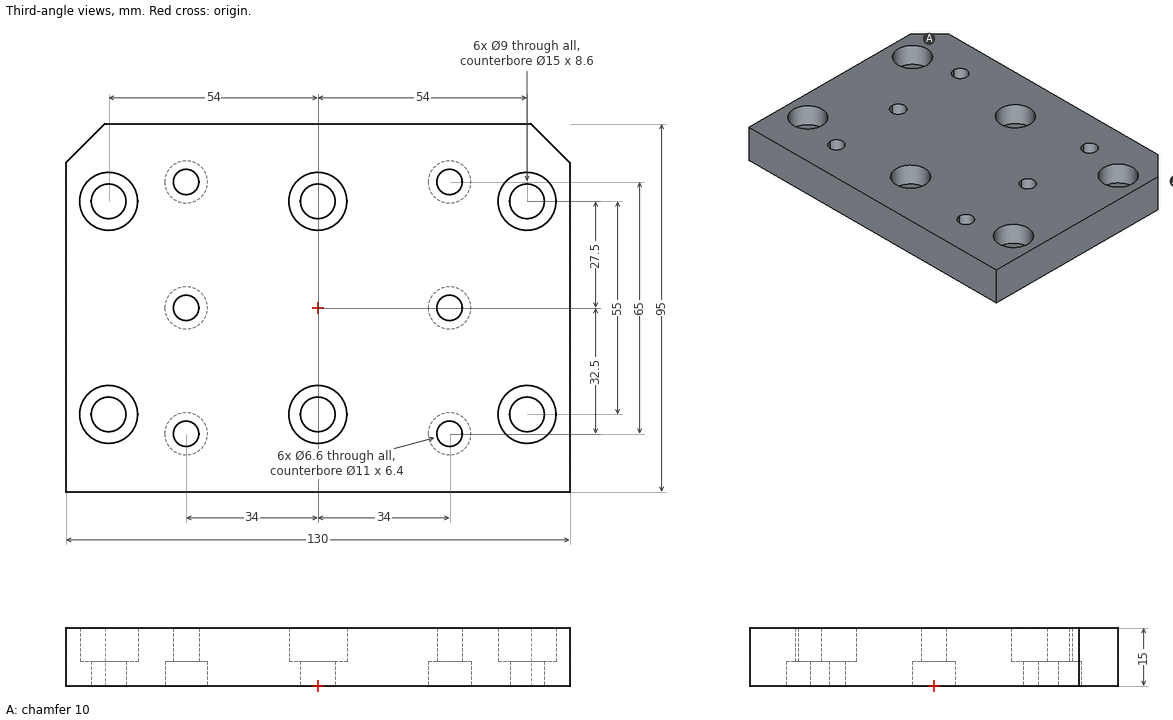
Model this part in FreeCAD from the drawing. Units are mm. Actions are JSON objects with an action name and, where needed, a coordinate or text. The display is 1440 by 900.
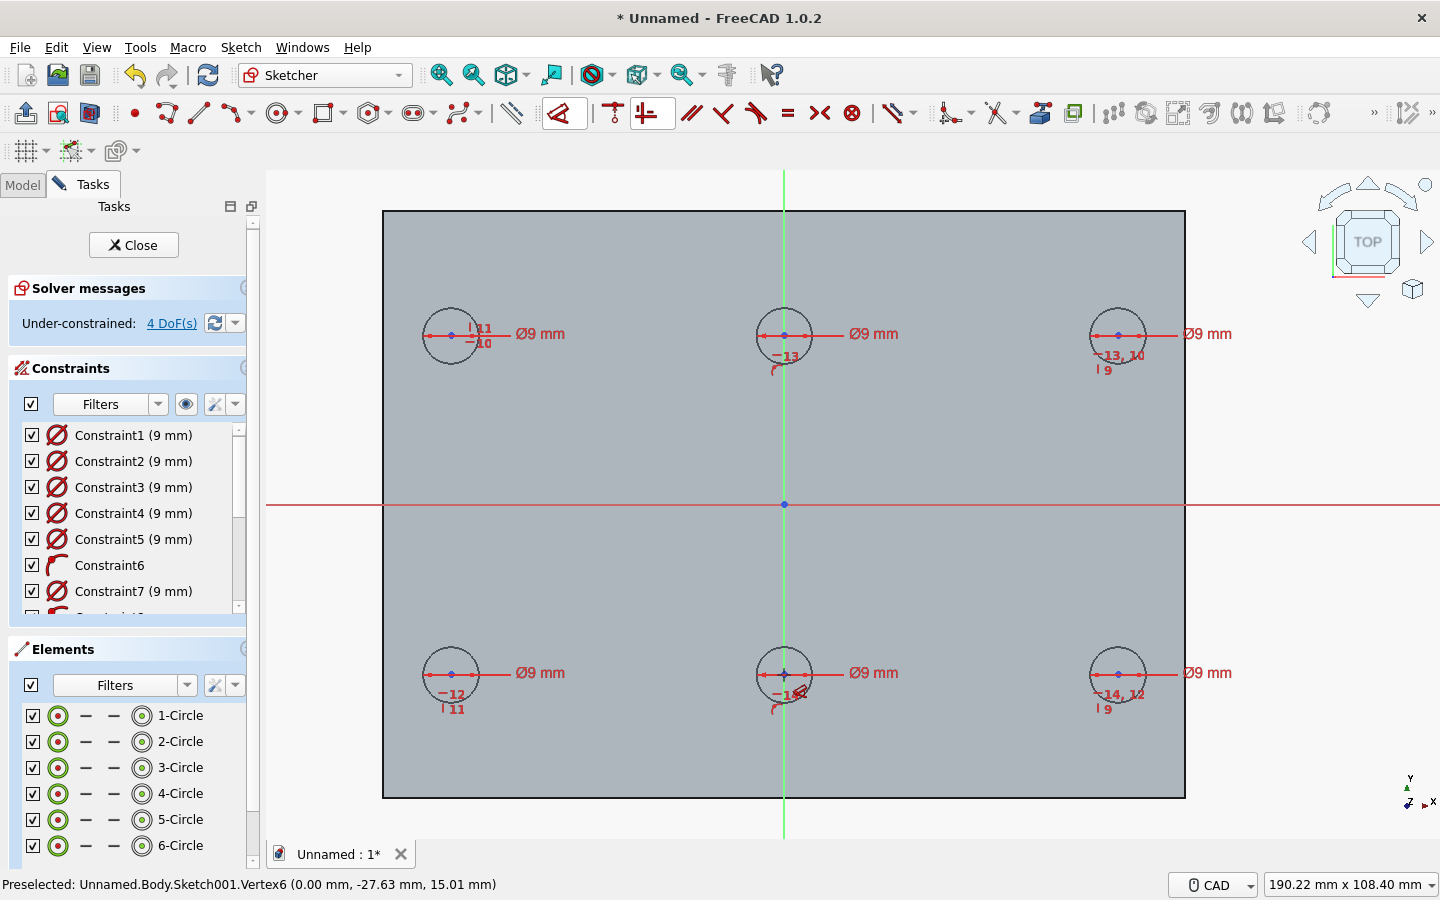
{"action": "left_click", "coordinate": [1118, 336]}
{"action": "left_click", "coordinate": [951, 302]}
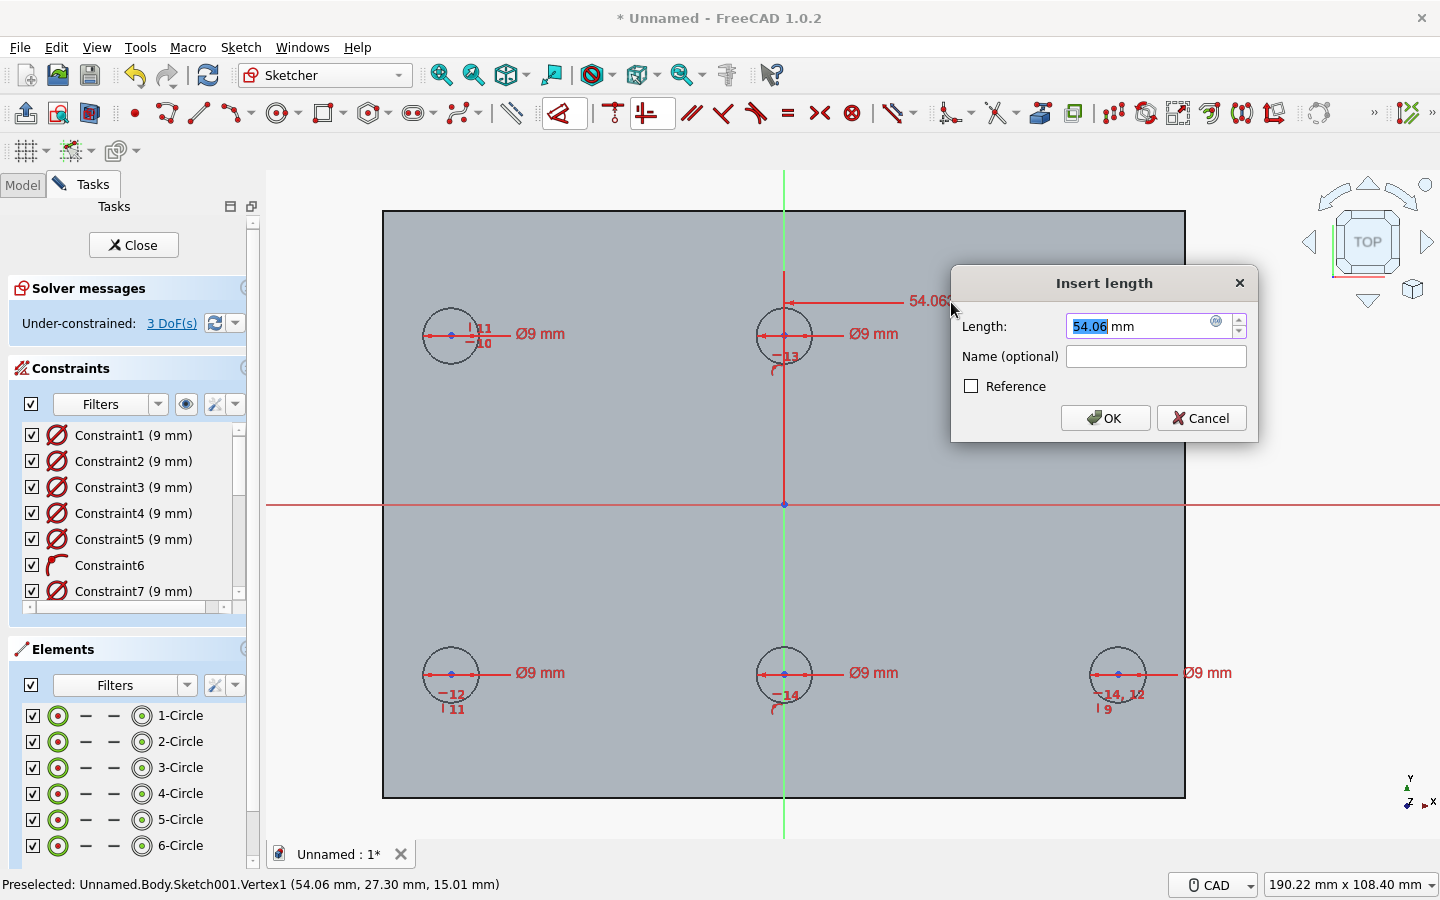
{"action": "type", "text": "54"}
{"action": "key", "text": "Return"}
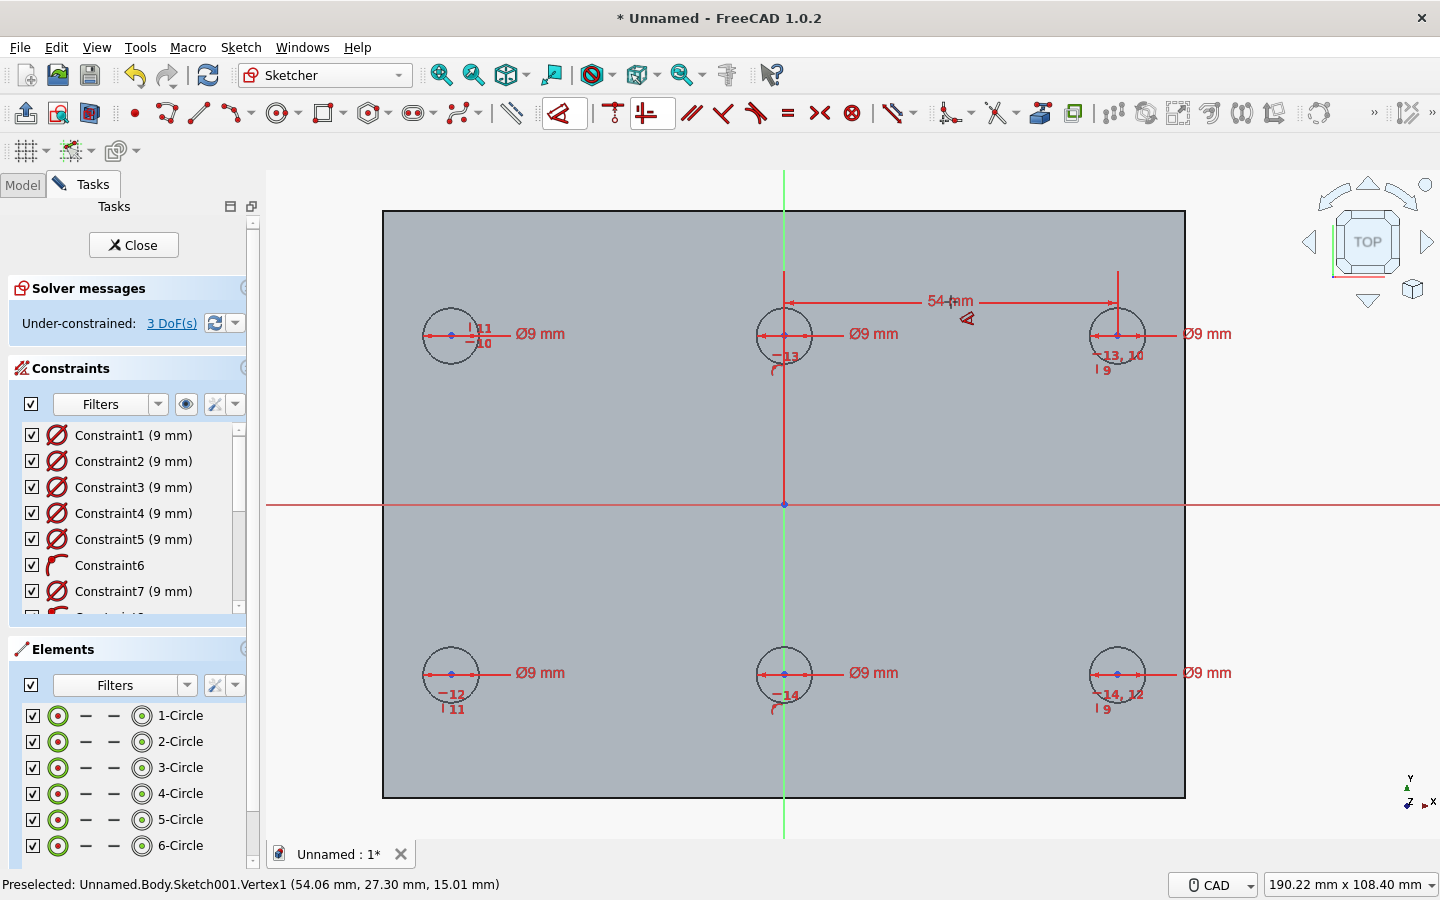
{"action": "left_click", "coordinate": [451, 336]}
{"action": "left_click", "coordinate": [618, 302]}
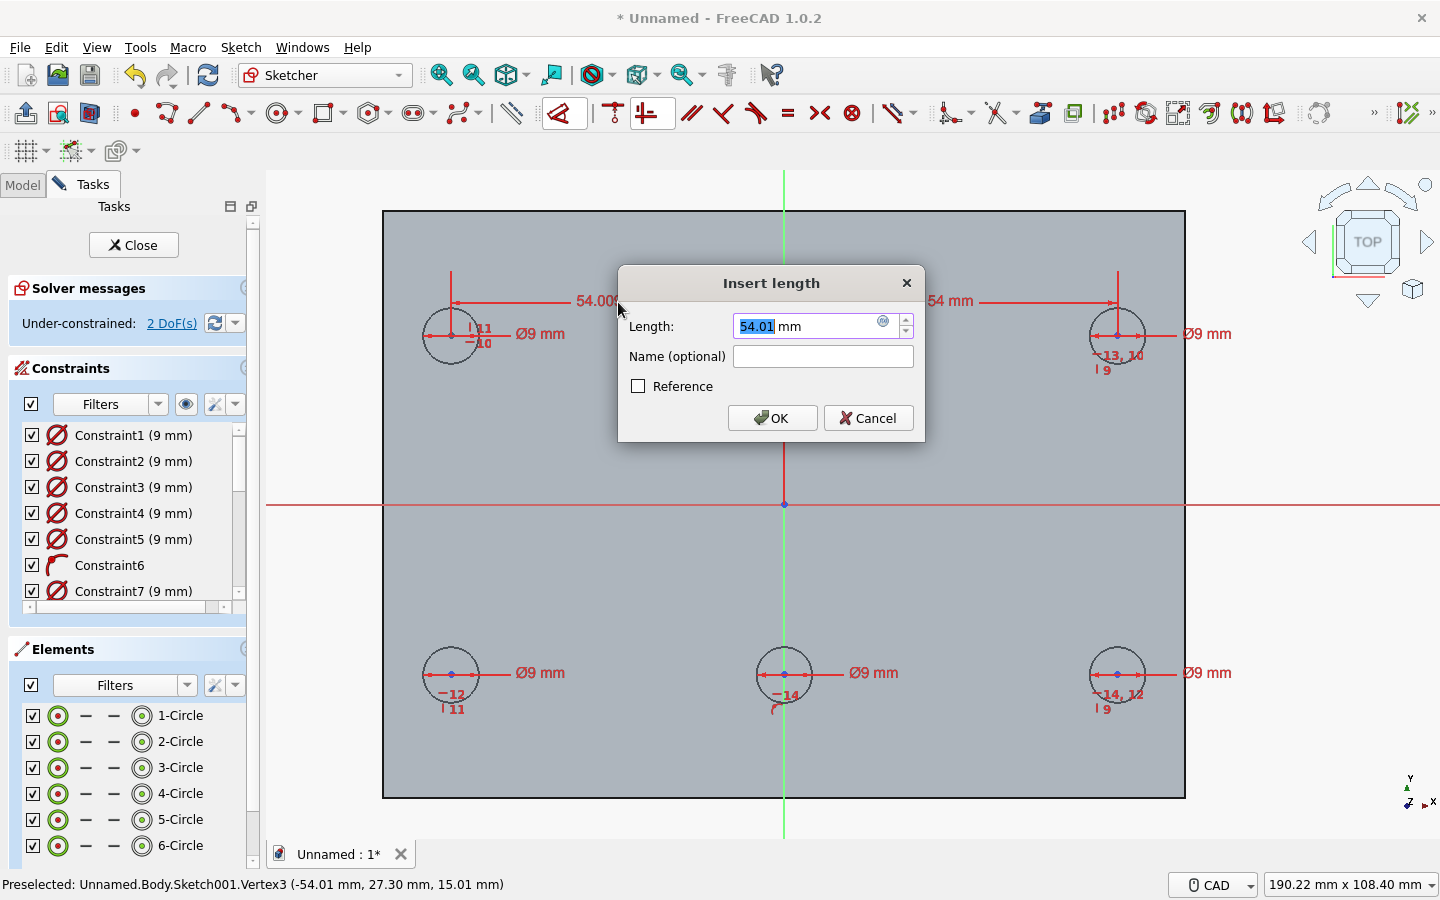
{"action": "type", "text": "54"}
{"action": "key", "text": "Return"}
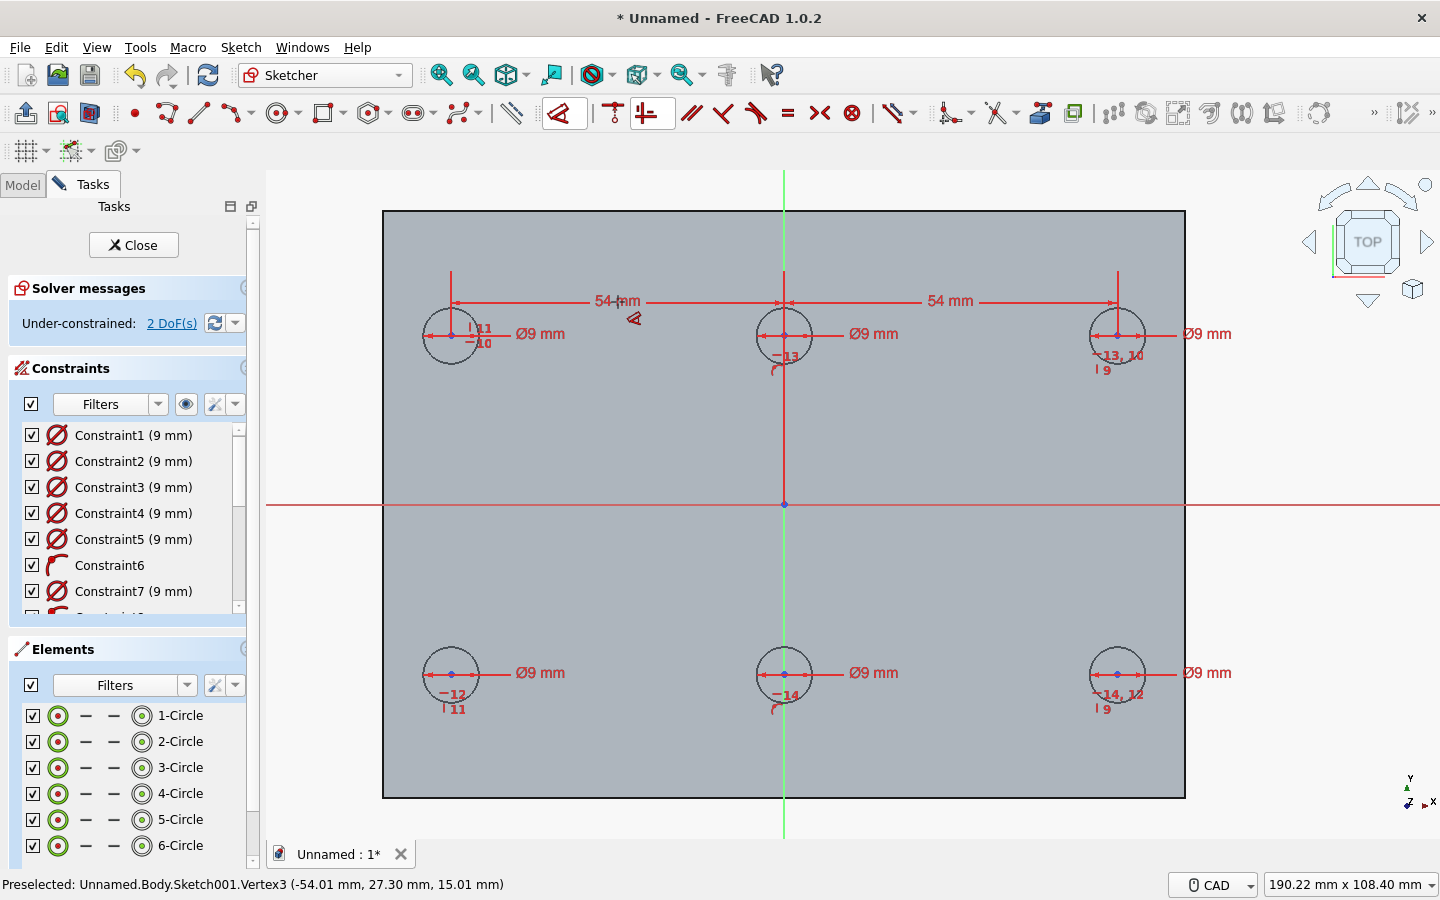
{"action": "left_click", "coordinate": [1118, 336]}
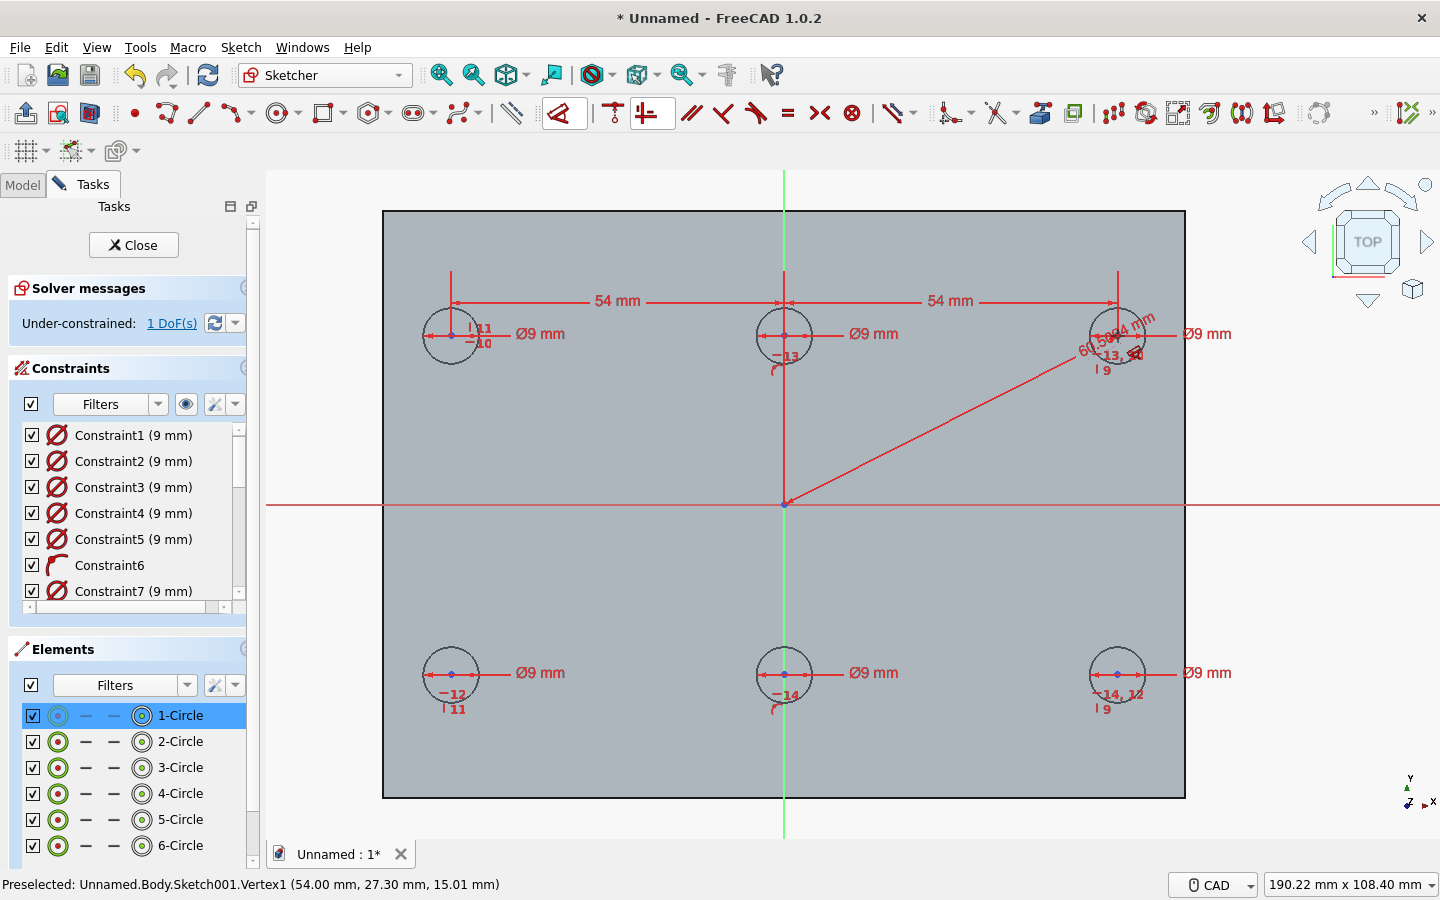
{"action": "left_click", "coordinate": [1118, 675]}
{"action": "left_click", "coordinate": [1152, 428]}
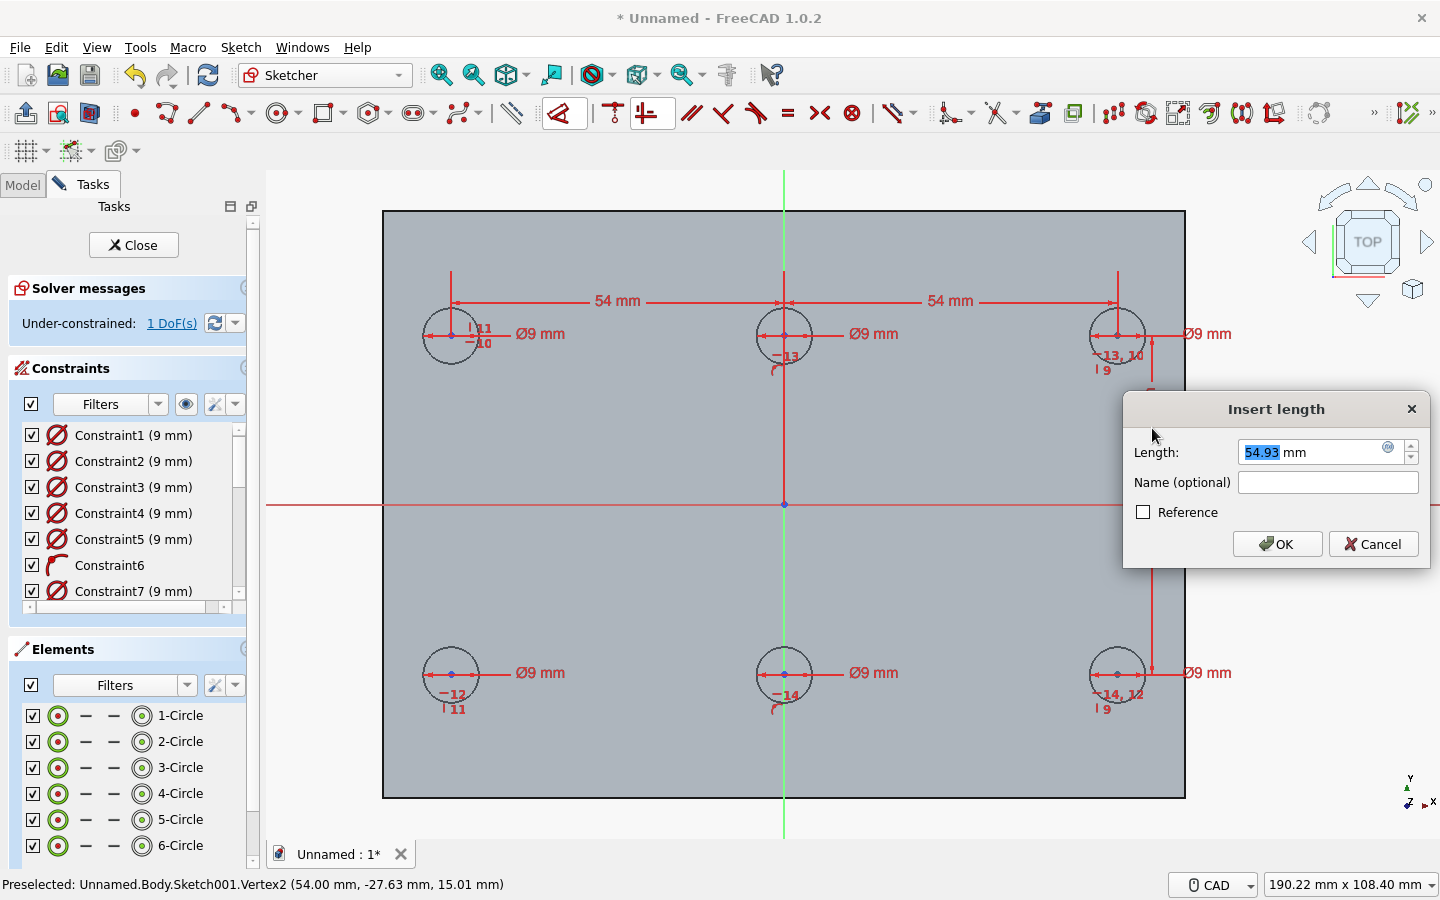
{"action": "type", "text": "55"}
{"action": "key", "text": "Return"}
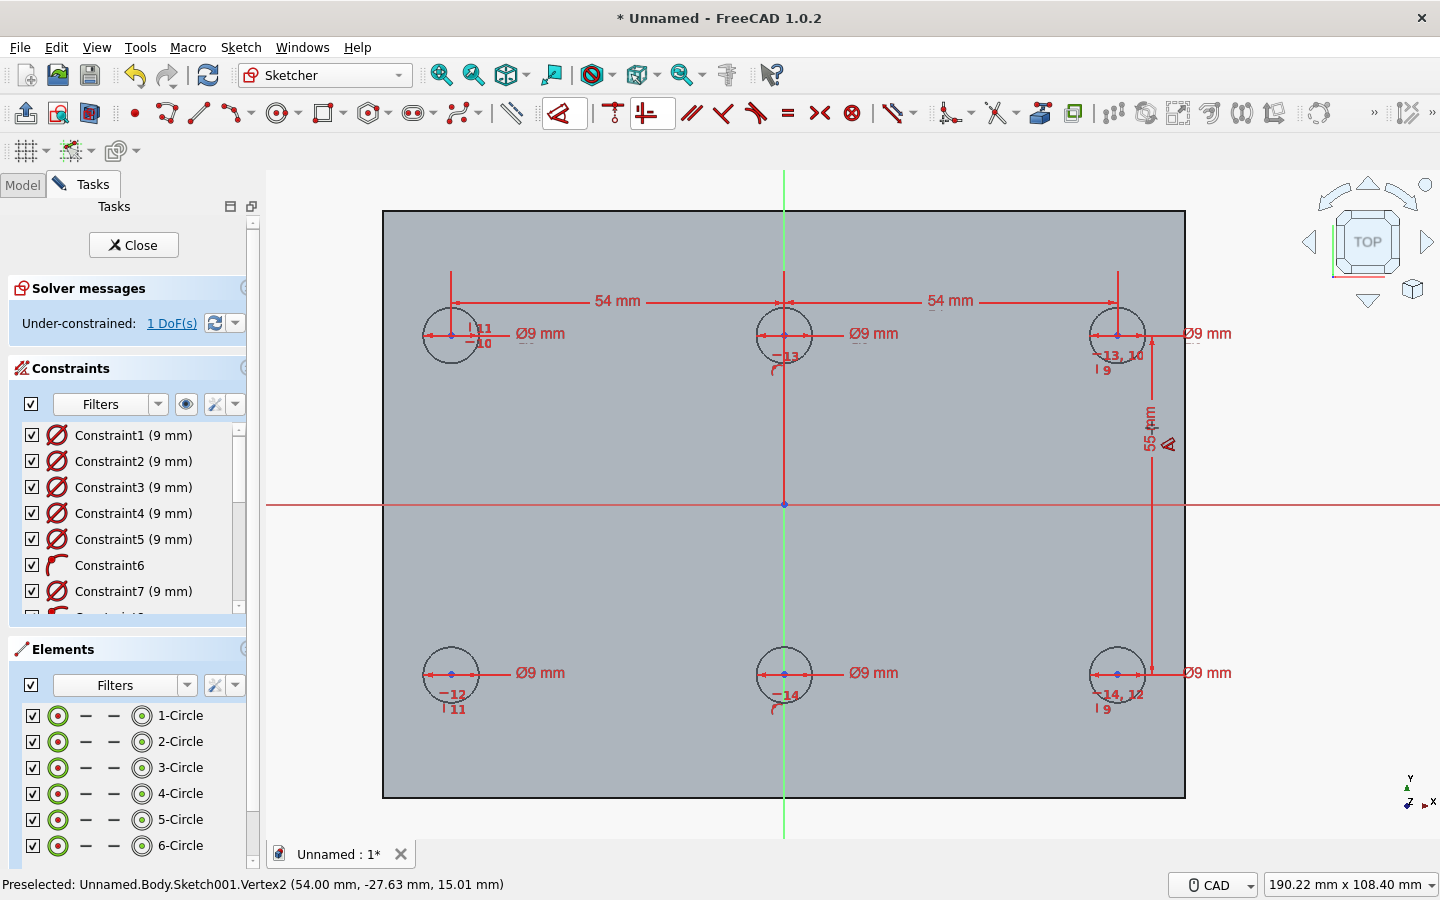
{"action": "left_click", "coordinate": [1118, 336]}
{"action": "left_click", "coordinate": [1152, 381]}